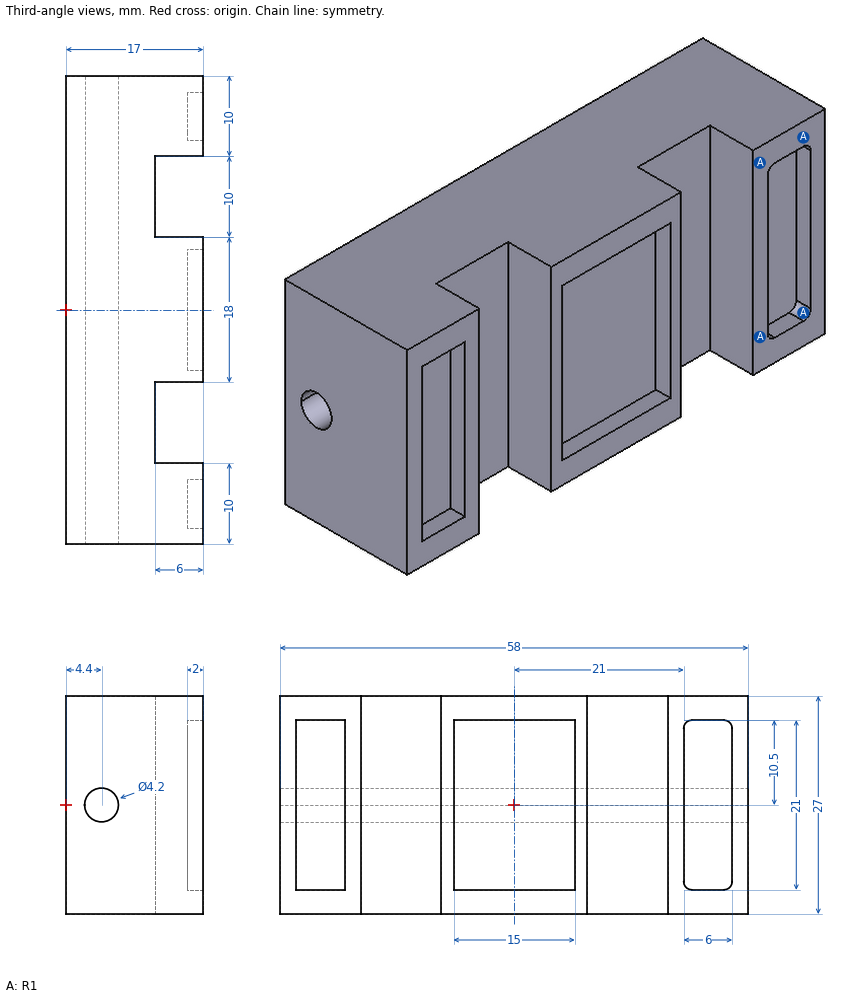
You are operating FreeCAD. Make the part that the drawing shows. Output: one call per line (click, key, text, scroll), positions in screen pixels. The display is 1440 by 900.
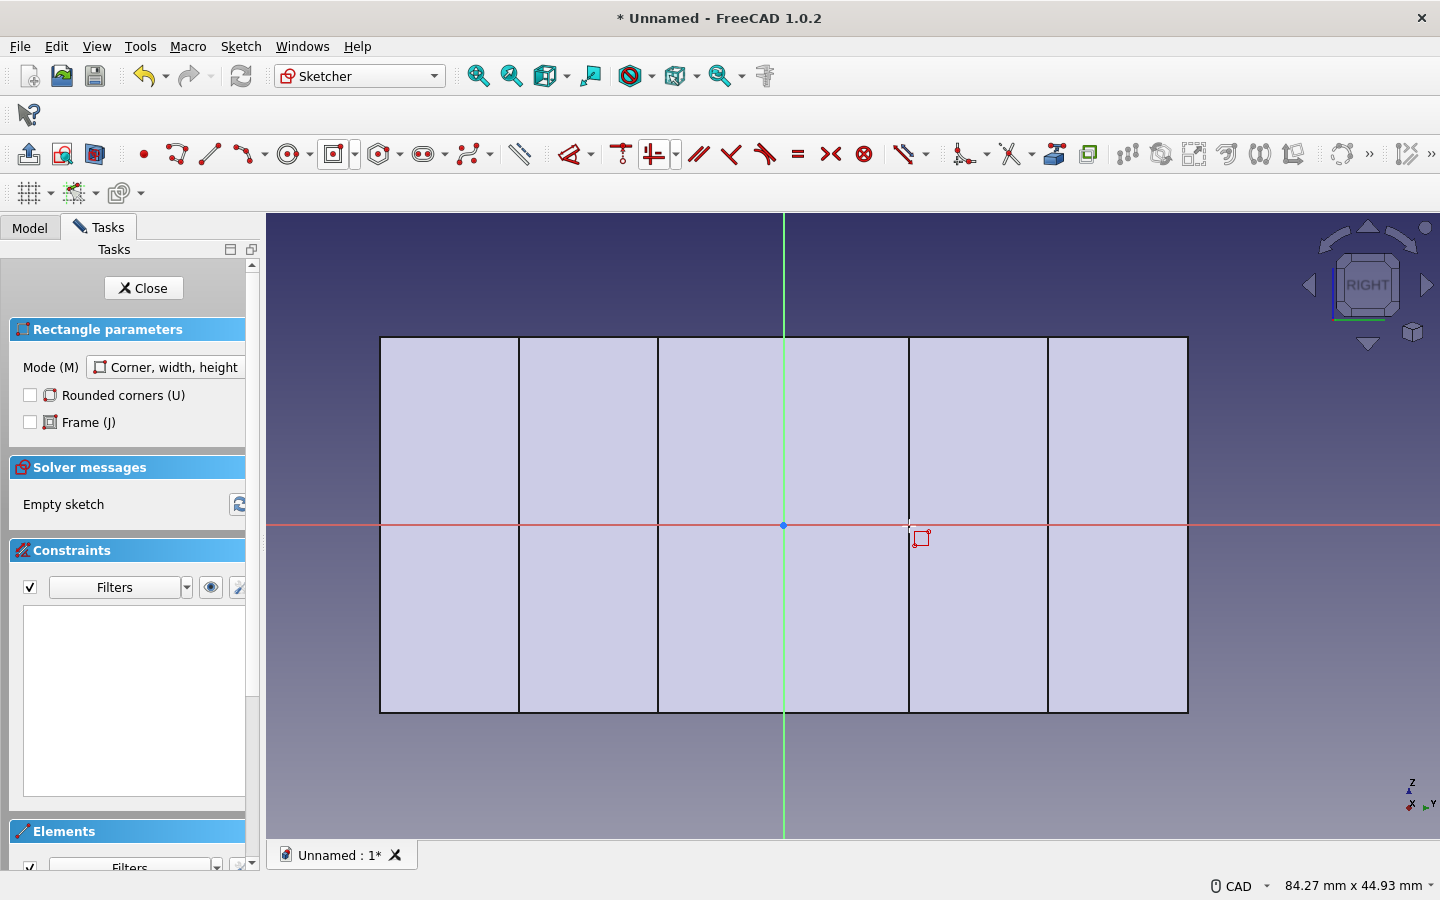
click(1076, 379)
click(1160, 672)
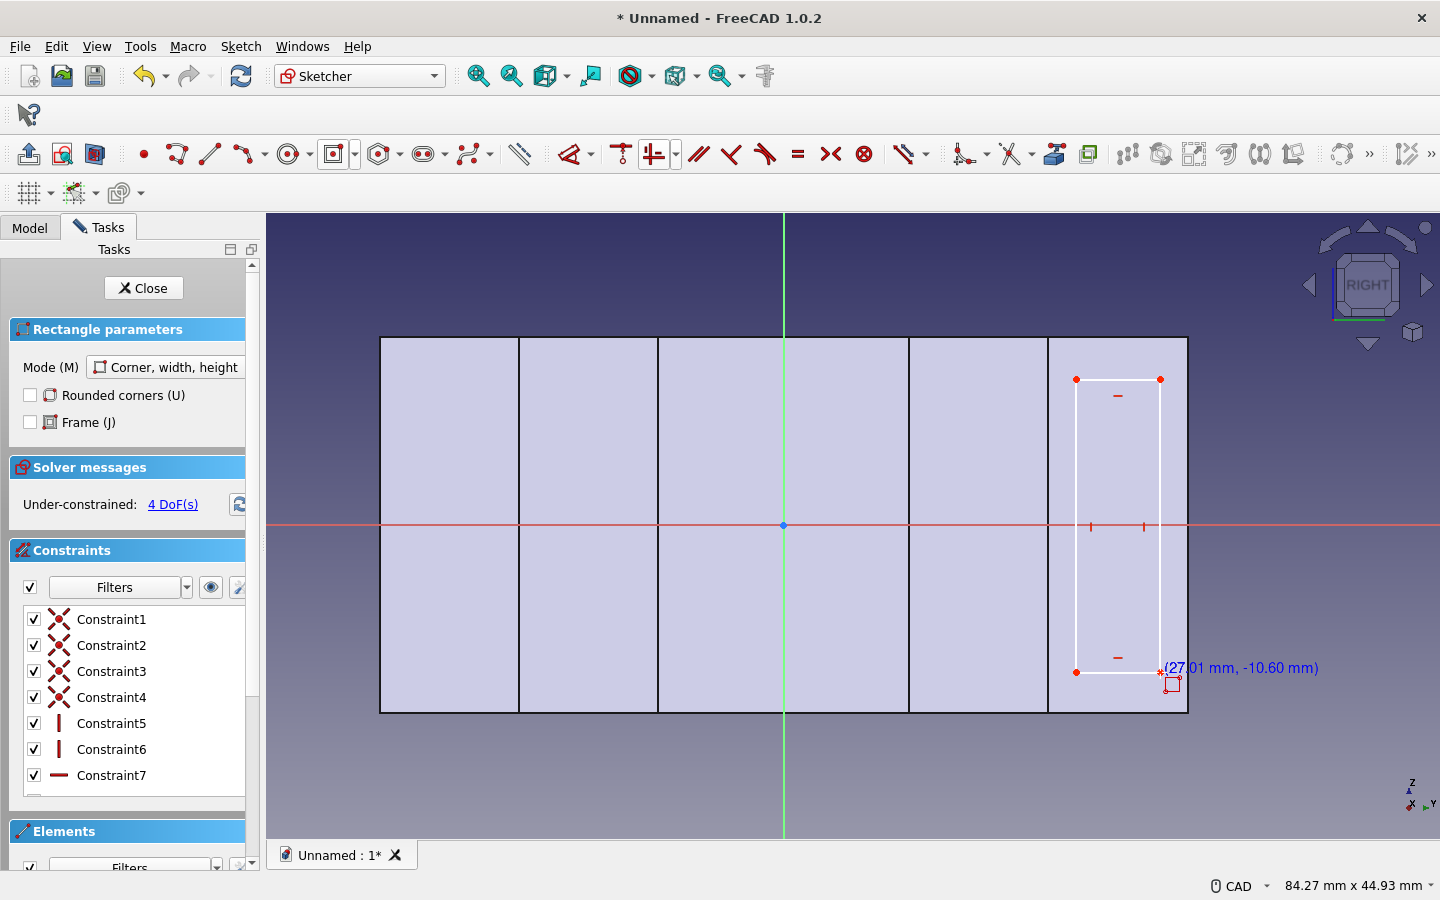
key(g)
key(v)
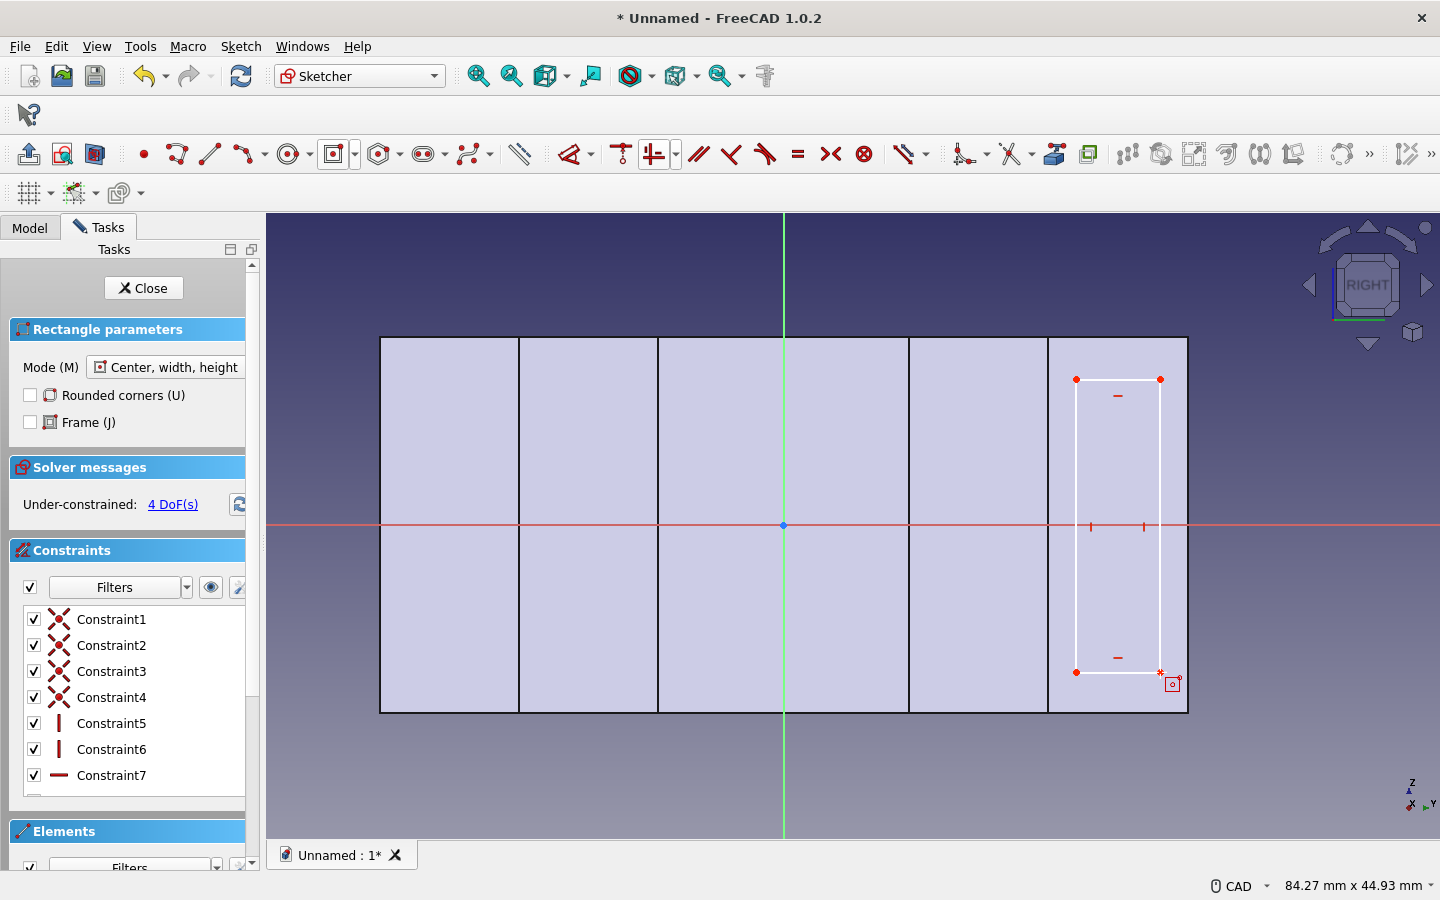
click(784, 525)
click(888, 379)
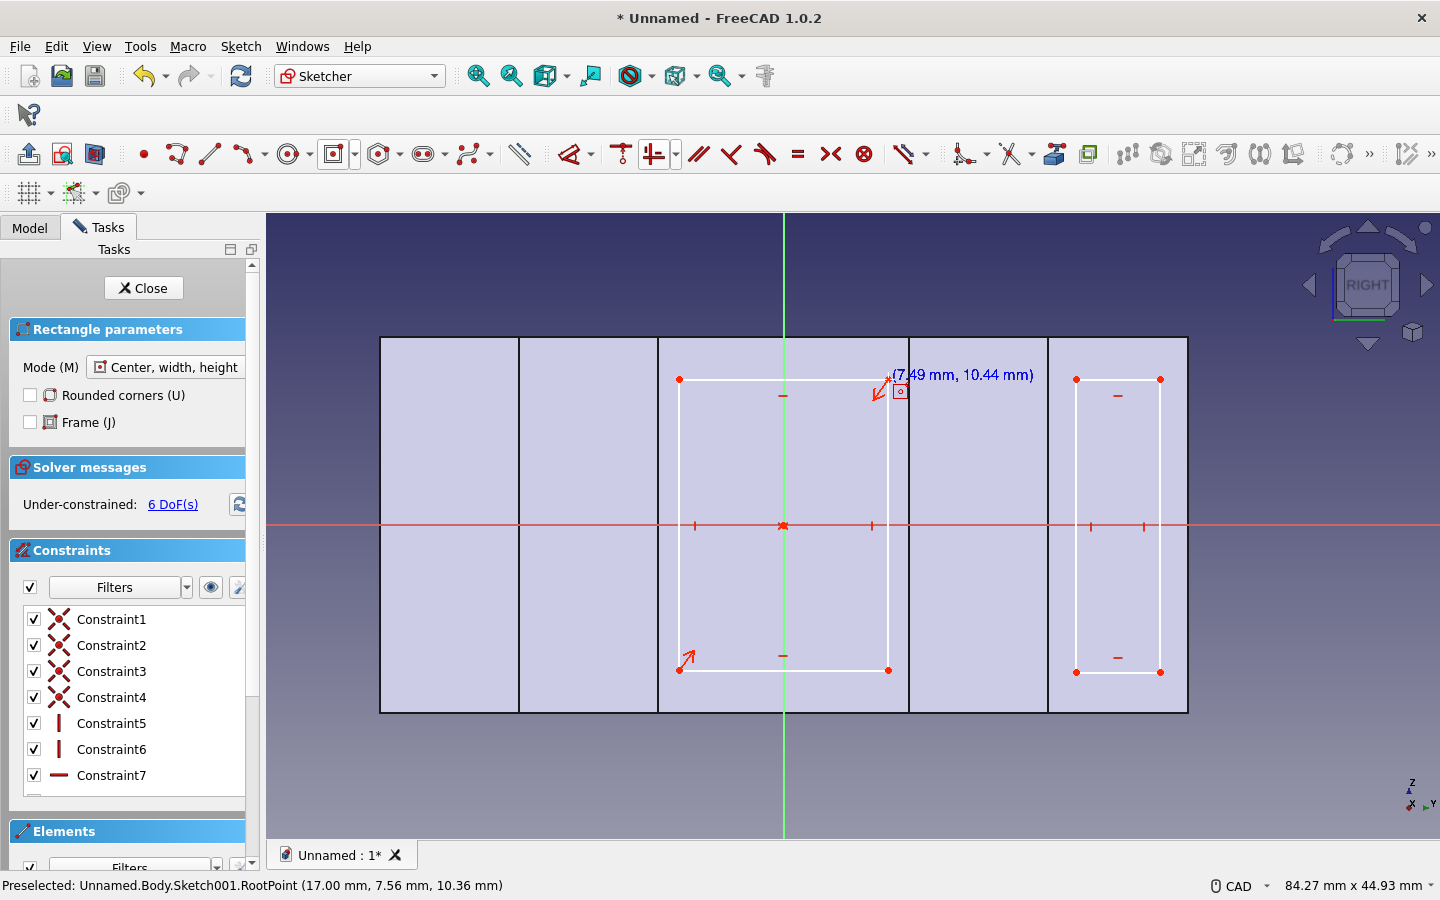
key(g)
key(r)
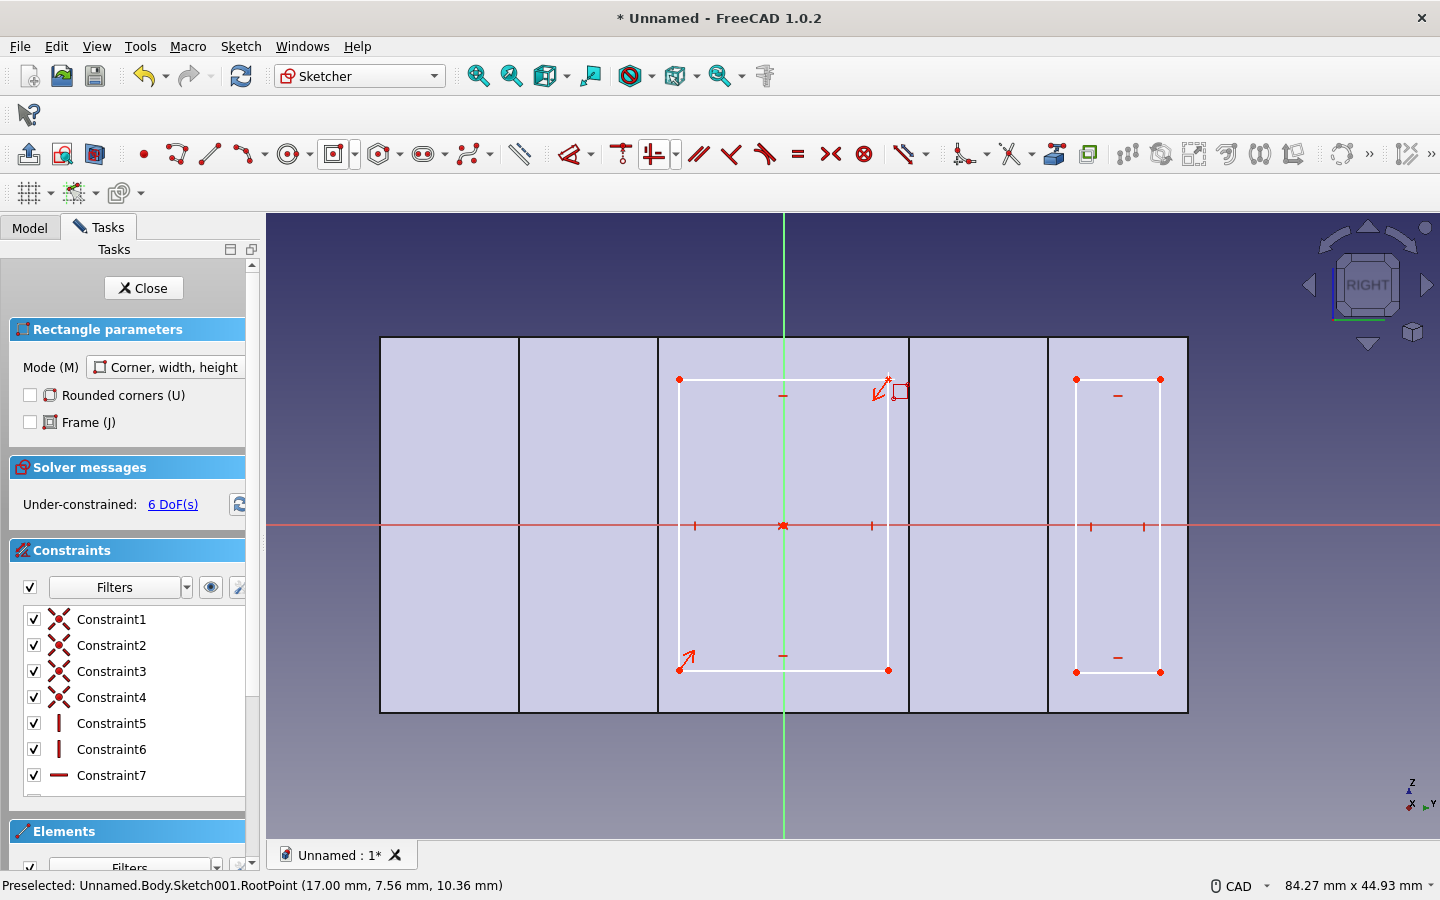
click(408, 379)
click(491, 672)
key(Escape)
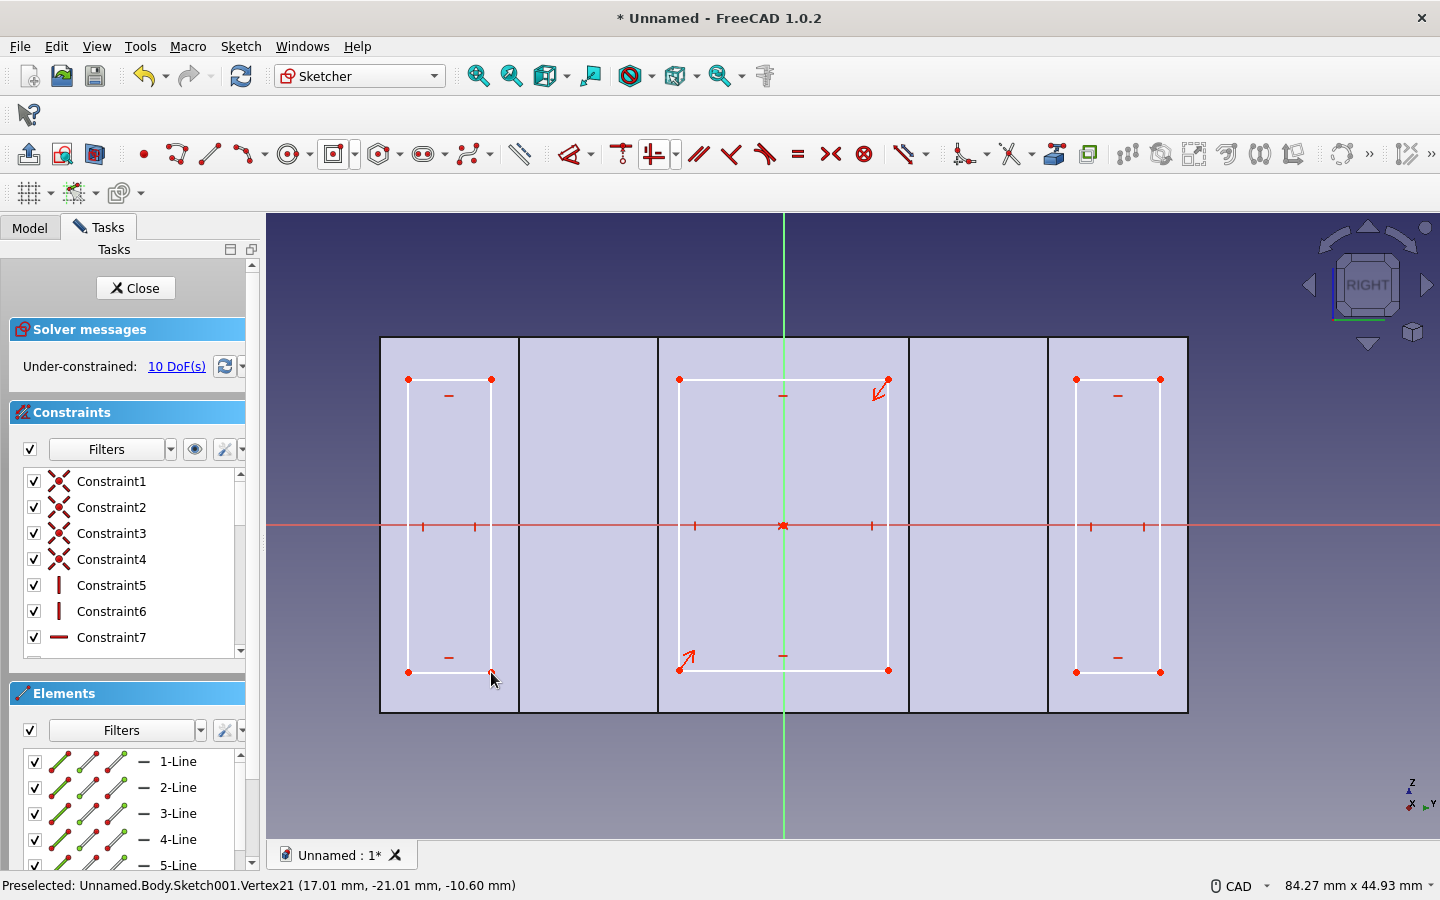
click(1160, 380)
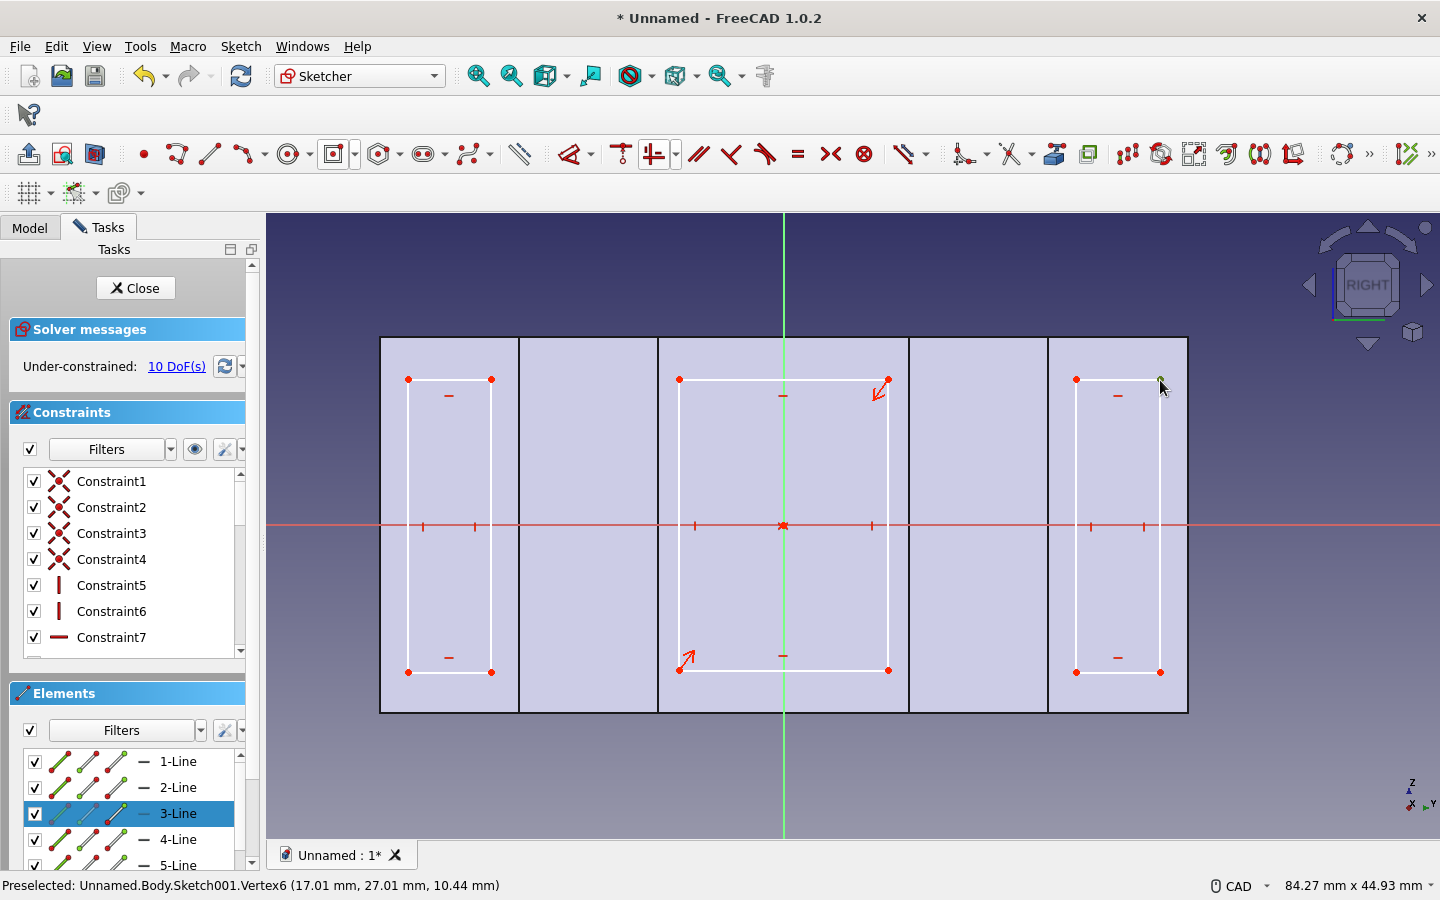
click(408, 380)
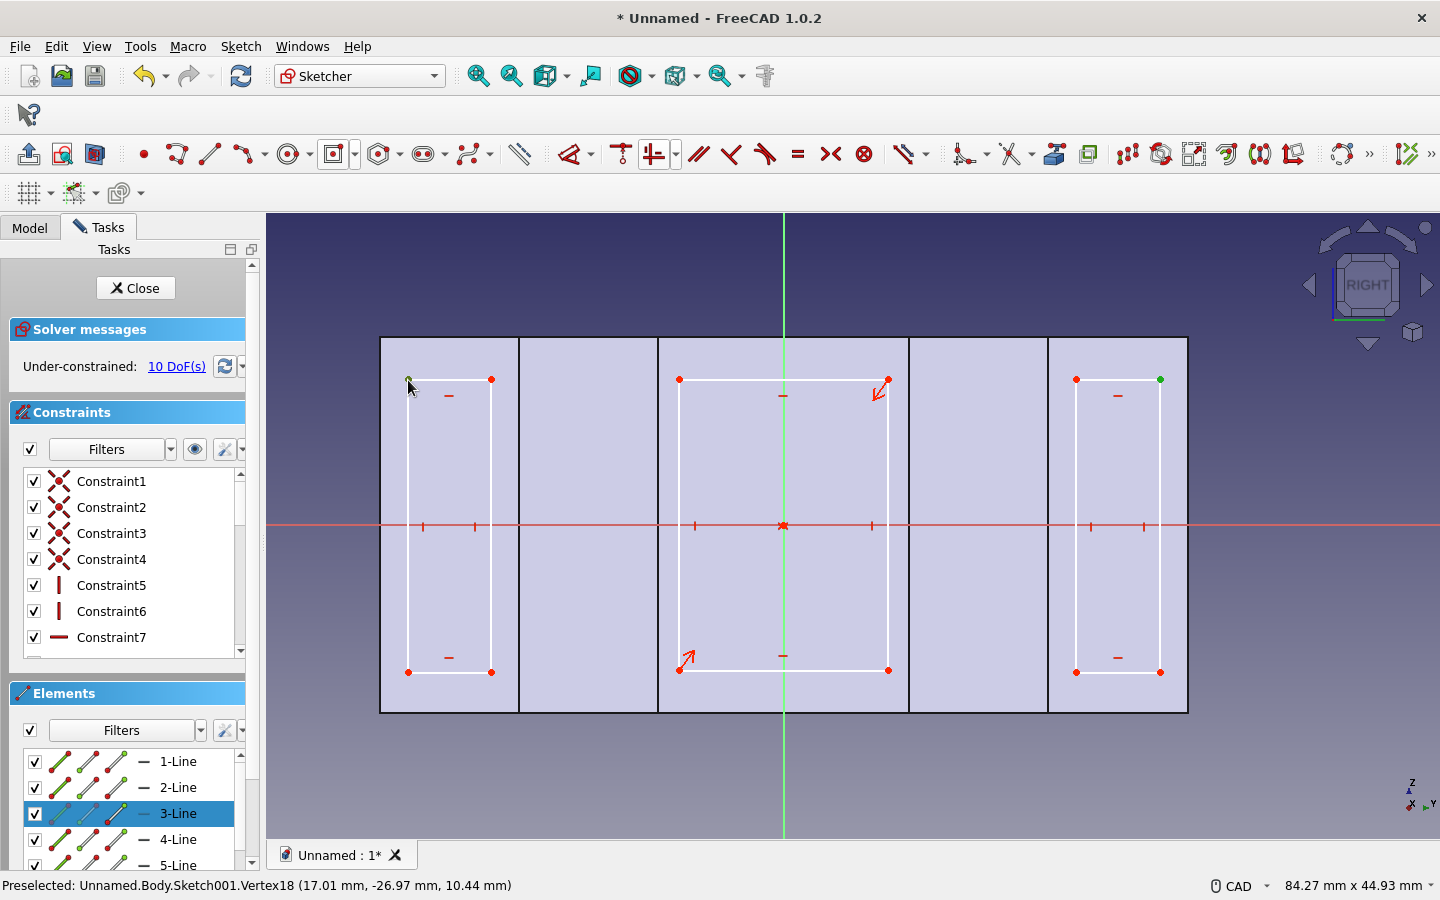
click(784, 770)